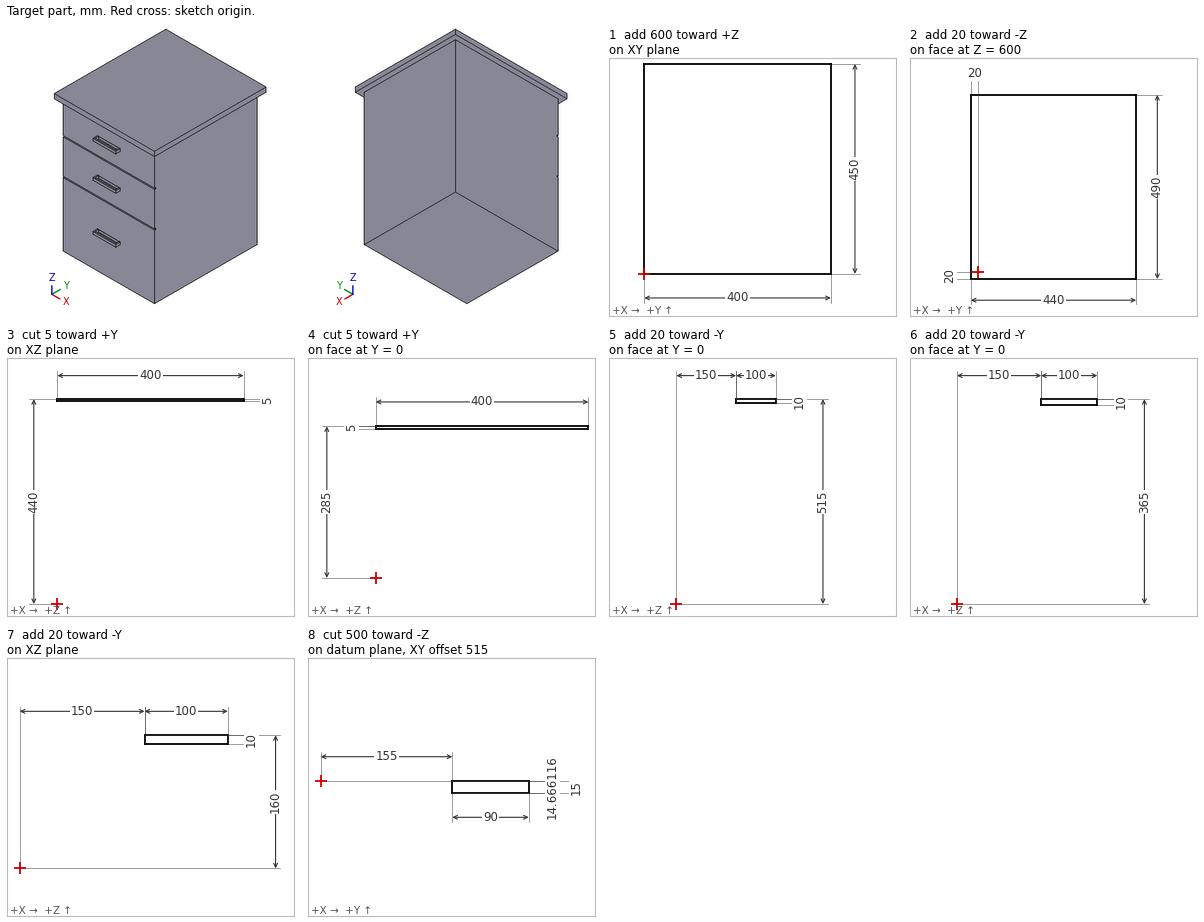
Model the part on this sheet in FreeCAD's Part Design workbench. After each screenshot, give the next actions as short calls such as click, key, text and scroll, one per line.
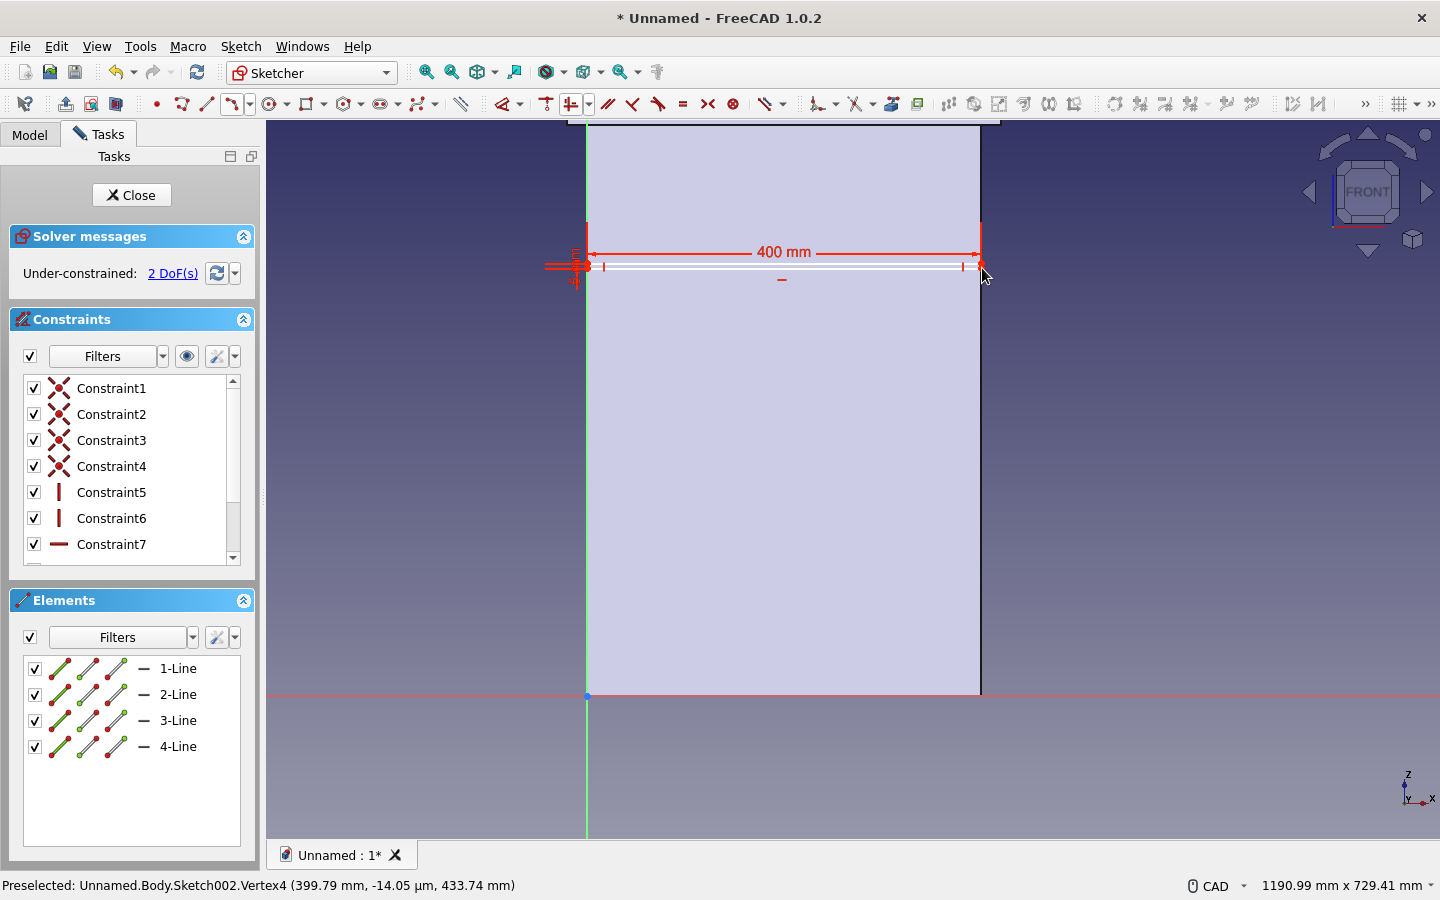
scroll(587, 264, up, 5)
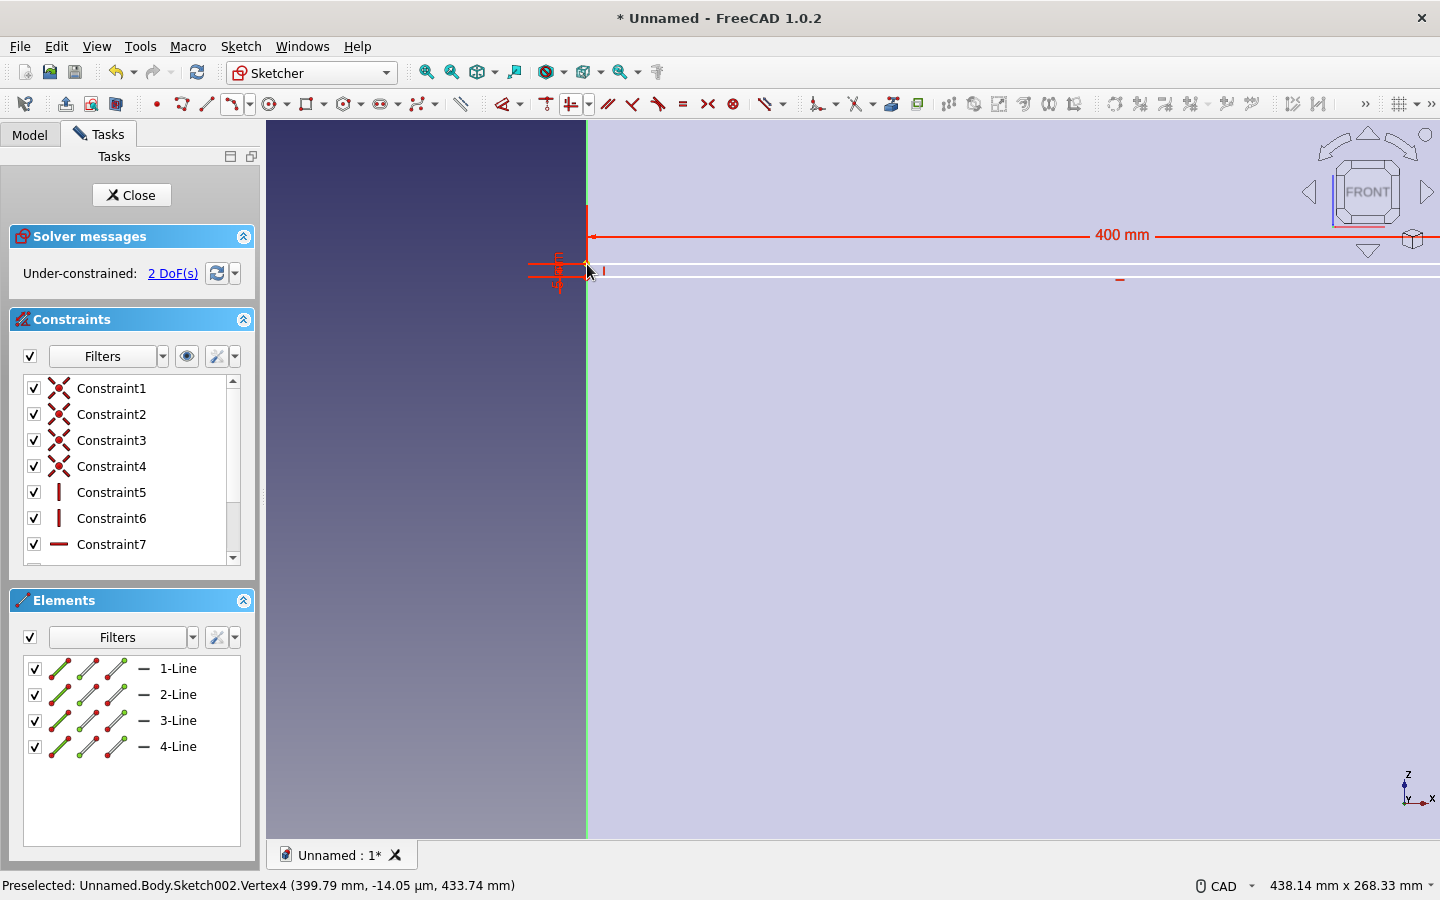
click(587, 264)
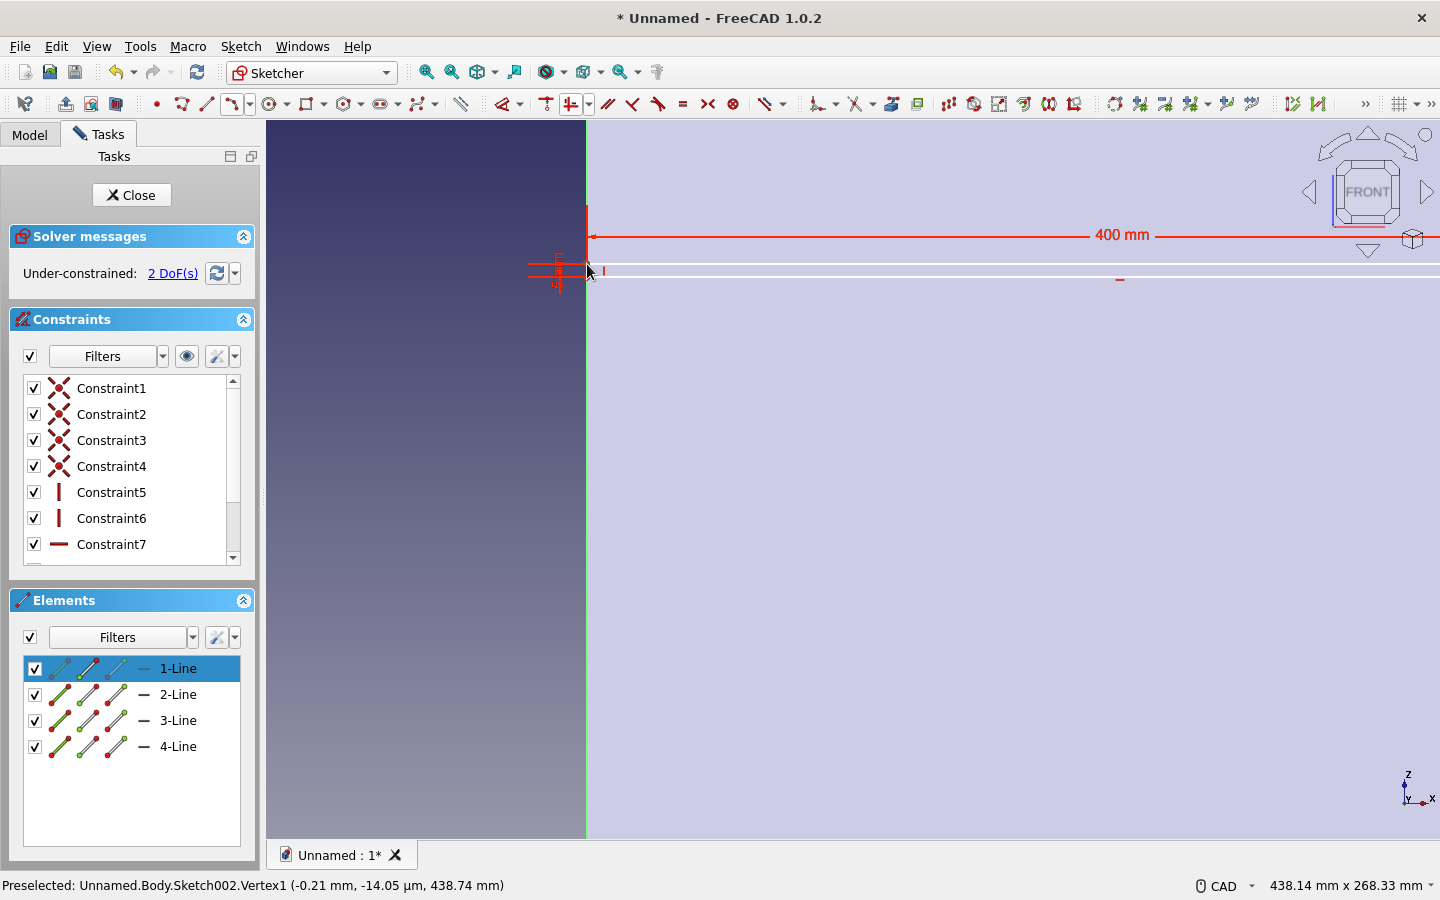
click(587, 764)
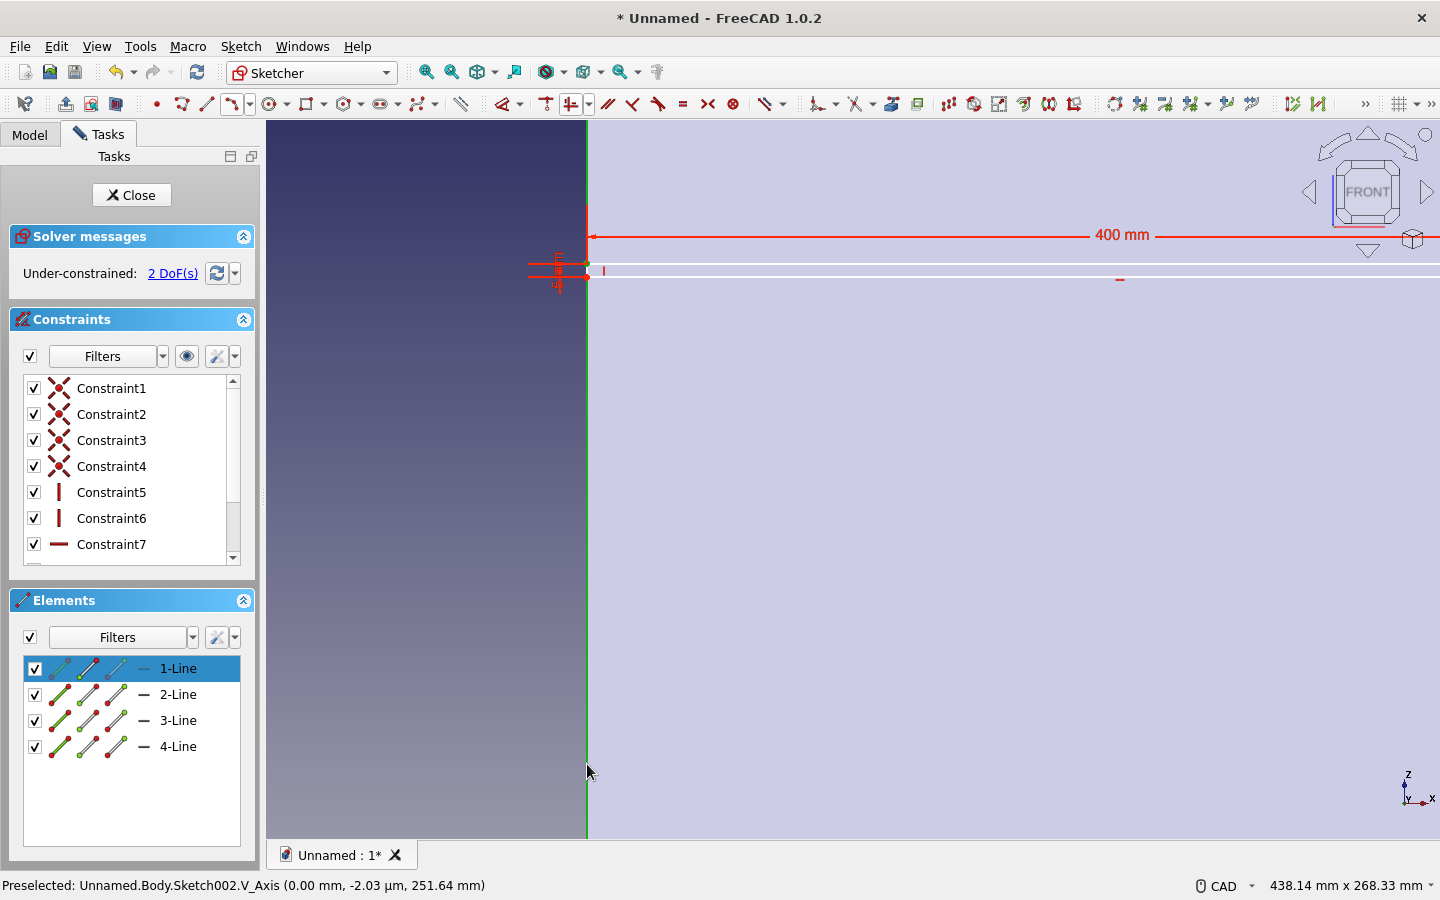
click(546, 104)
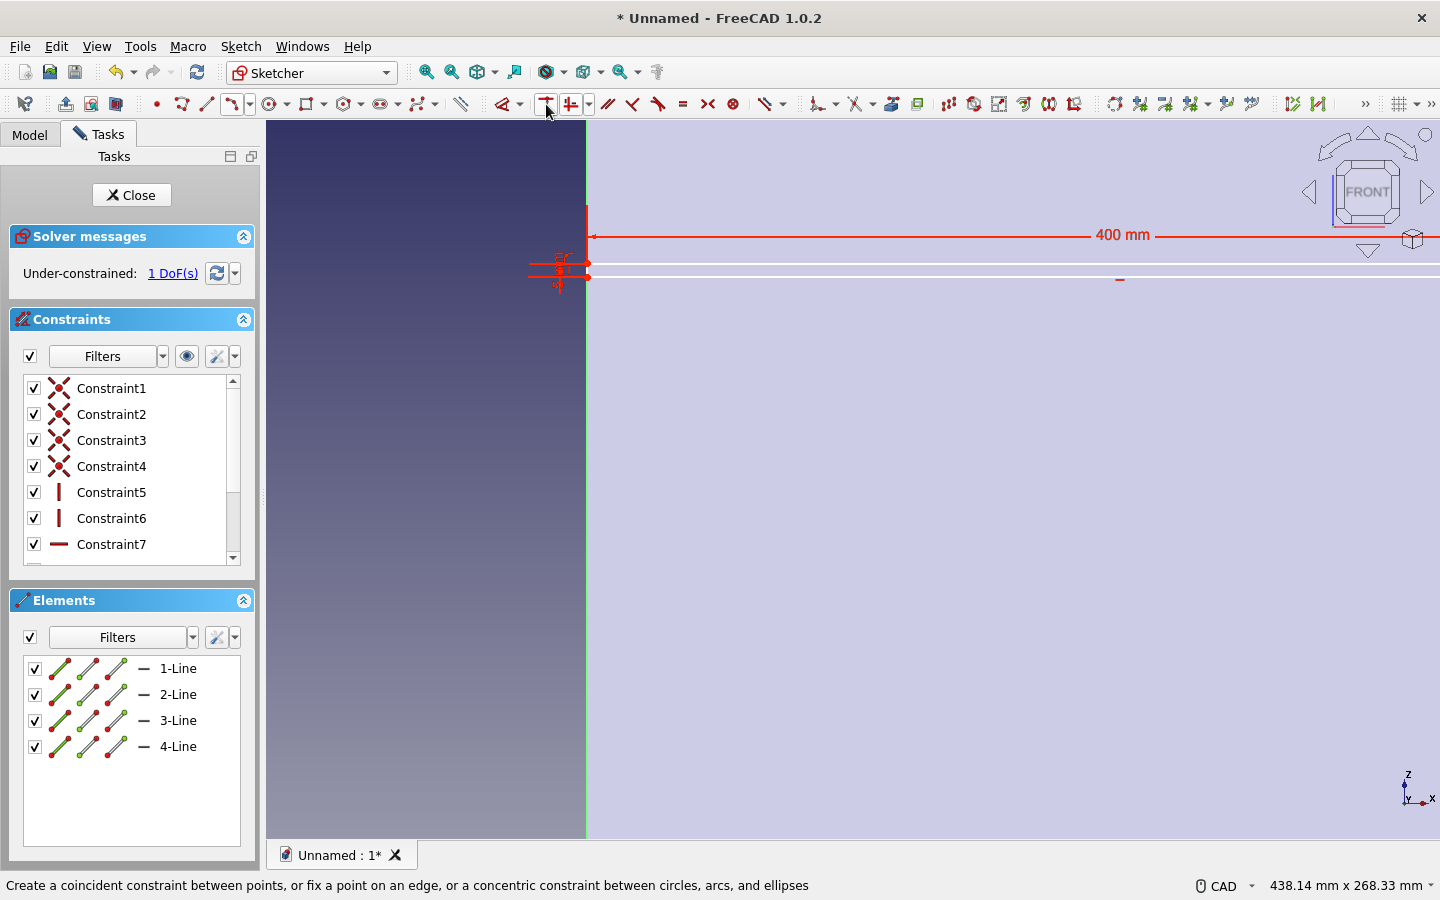
click(502, 104)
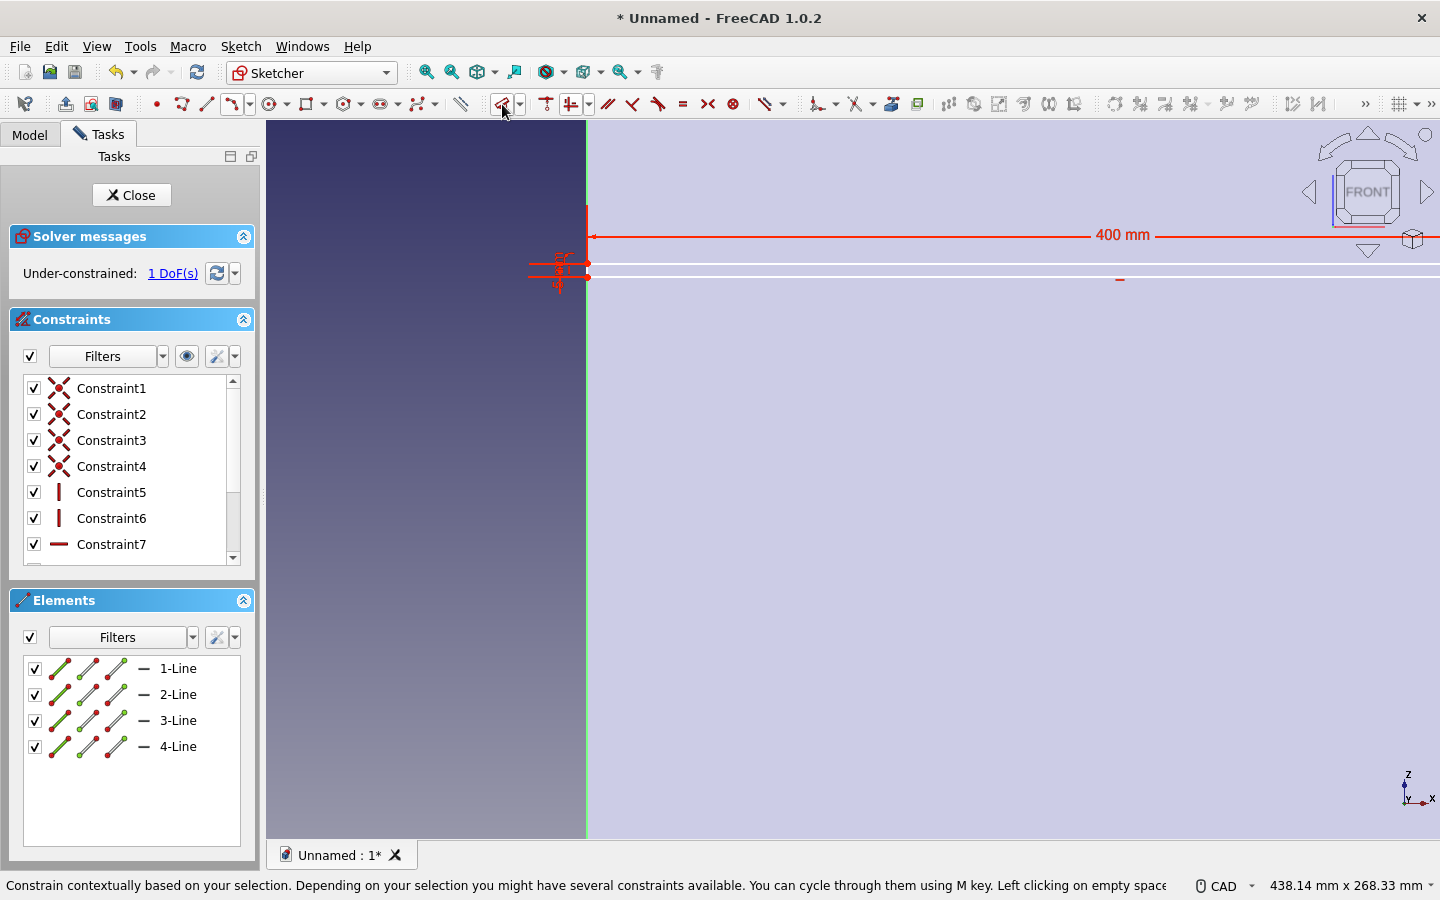
click(587, 264)
click(553, 537)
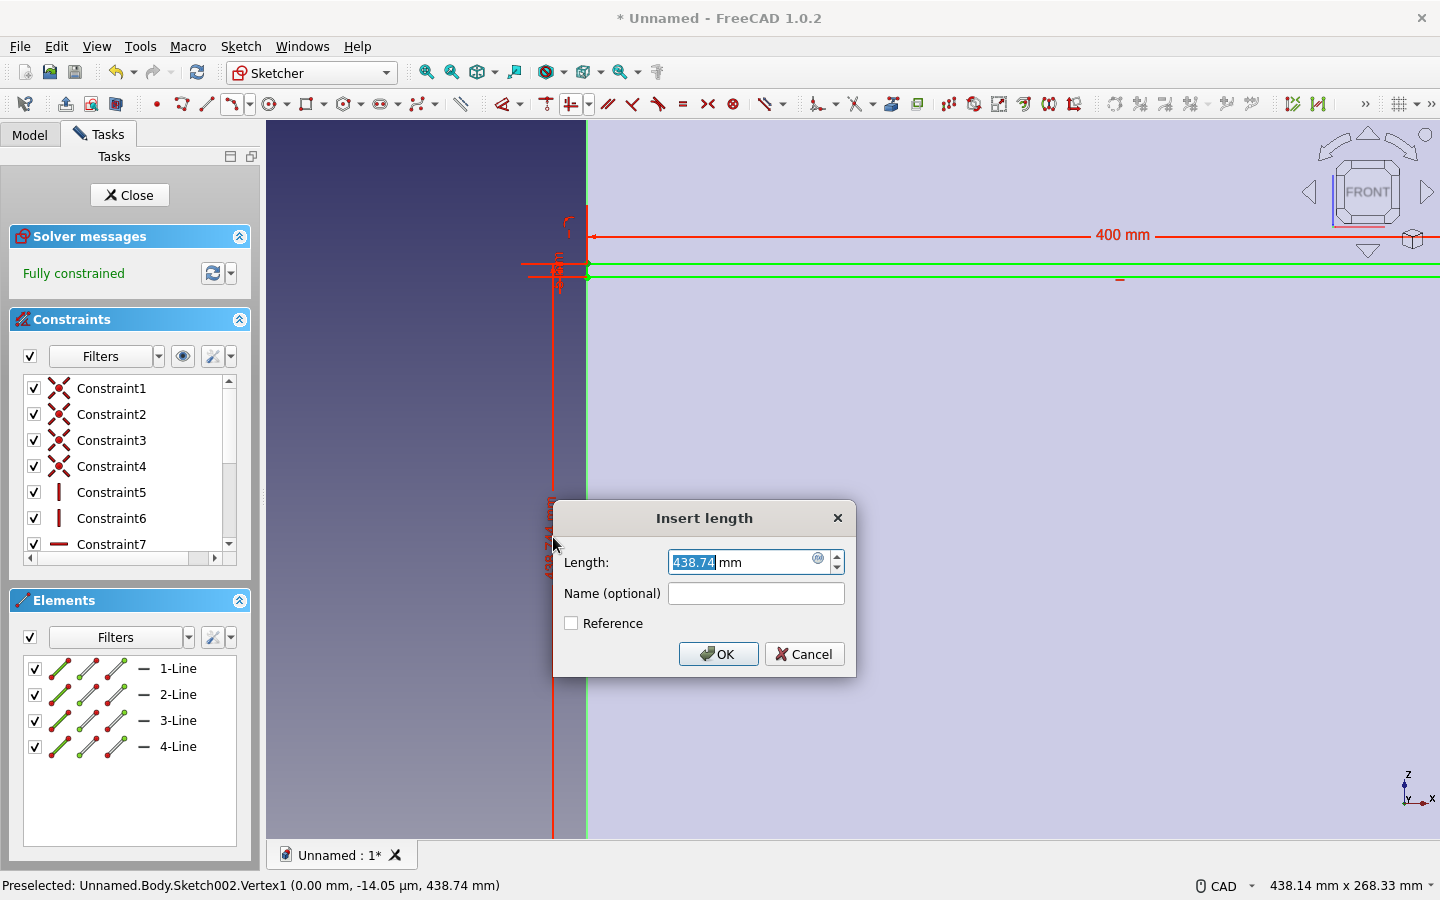
text(440)
key(Return)
key(Escape)